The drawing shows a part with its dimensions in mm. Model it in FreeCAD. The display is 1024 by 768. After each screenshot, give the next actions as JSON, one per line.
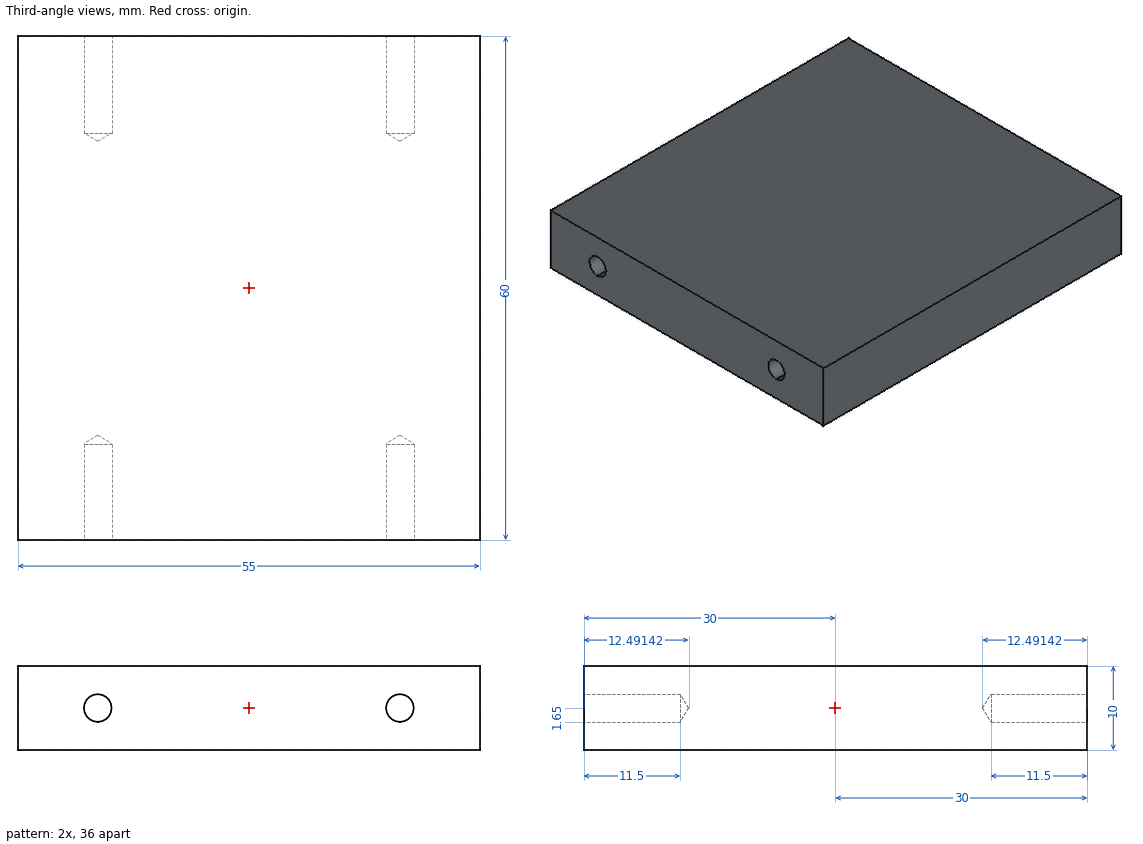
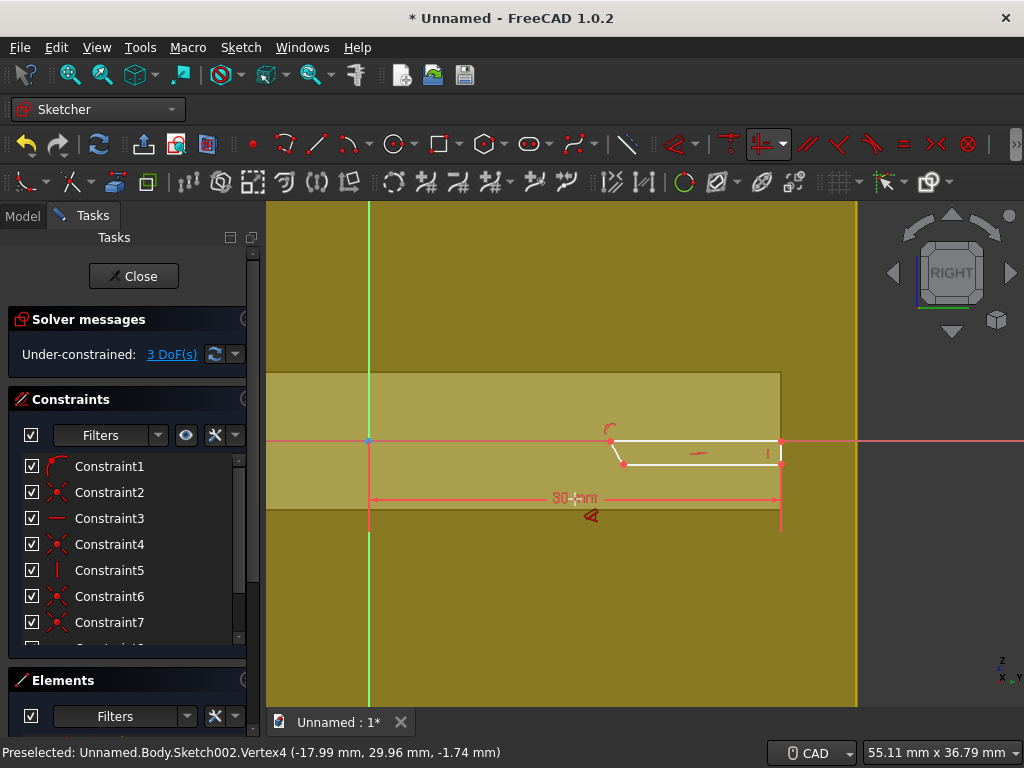
{"action": "left_click", "coordinate": [671, 465]}
{"action": "left_click", "coordinate": [702, 499]}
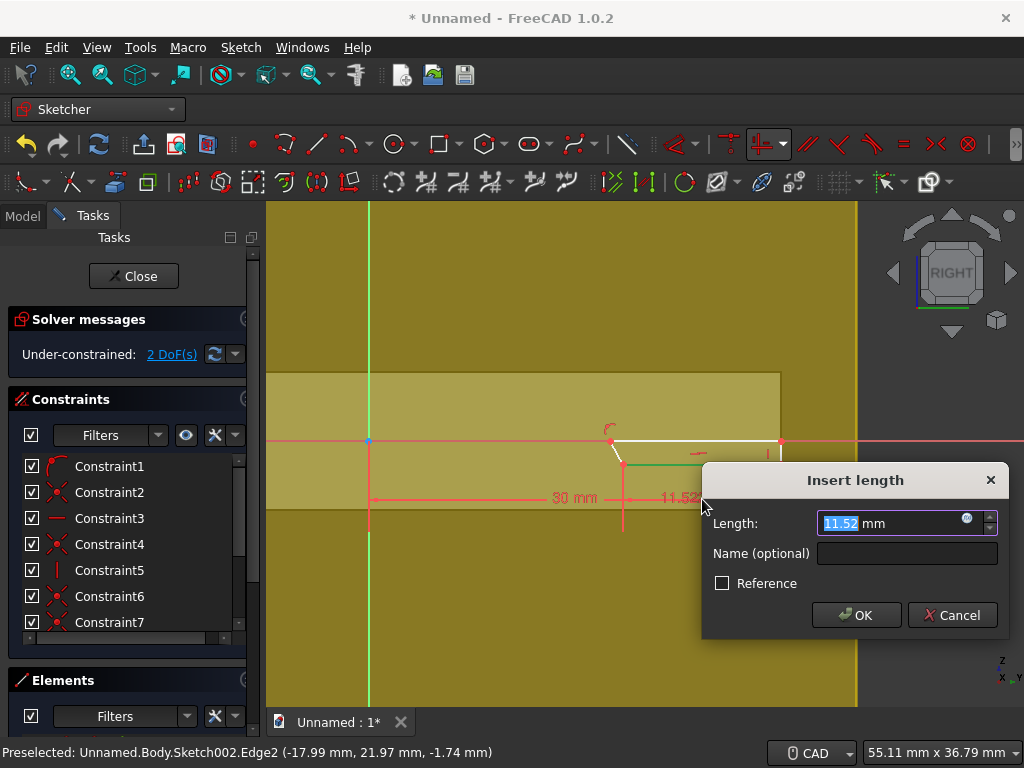
{"action": "type", "text": "11.5"}
{"action": "key", "text": "Return"}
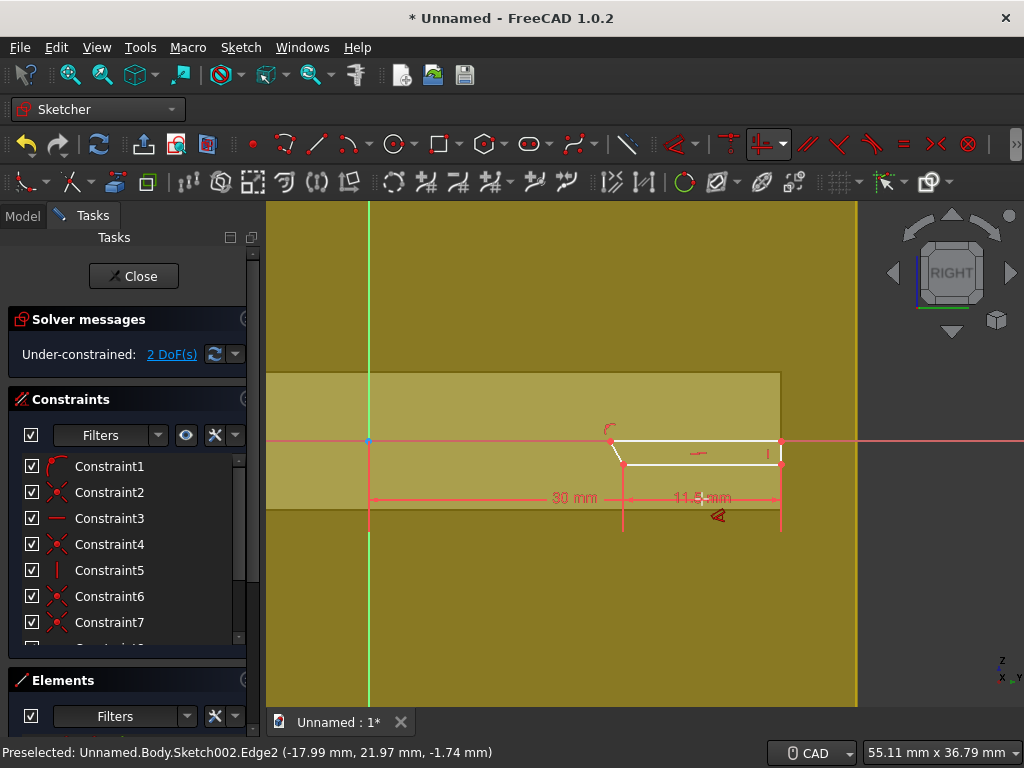
{"action": "scroll", "coordinate": [781, 455], "scroll_direction": "up", "scroll_amount": 3}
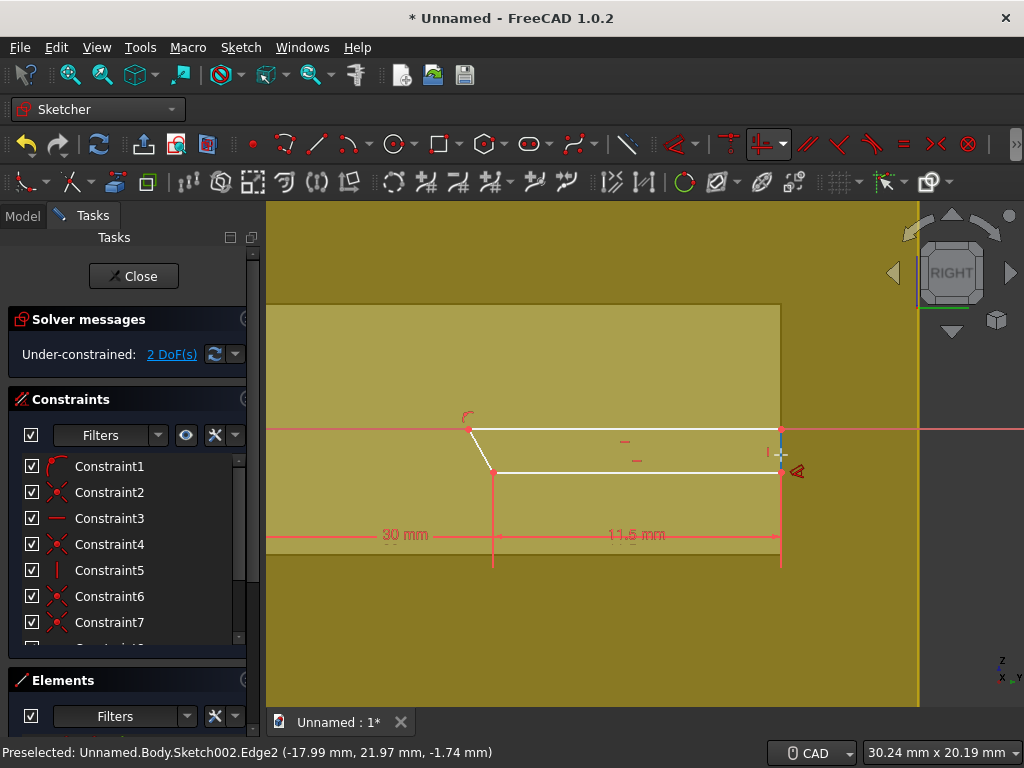
{"action": "left_click", "coordinate": [781, 455]}
{"action": "left_click", "coordinate": [815, 451]}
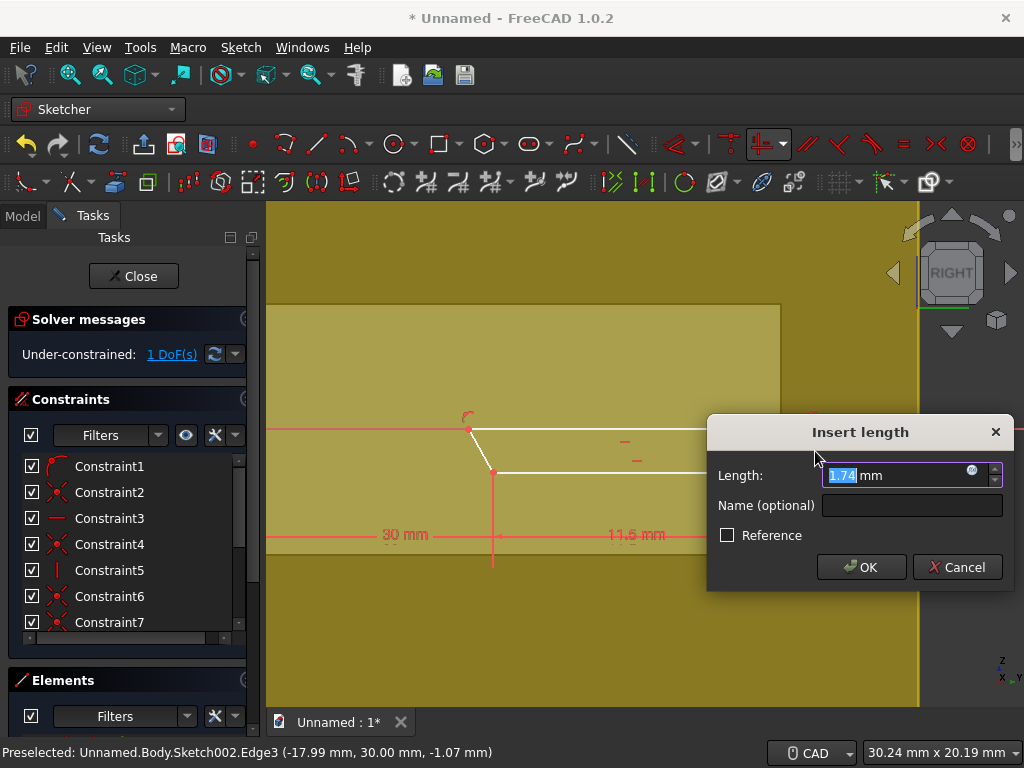
{"action": "type", "text": "1.65"}
{"action": "key", "text": "Return"}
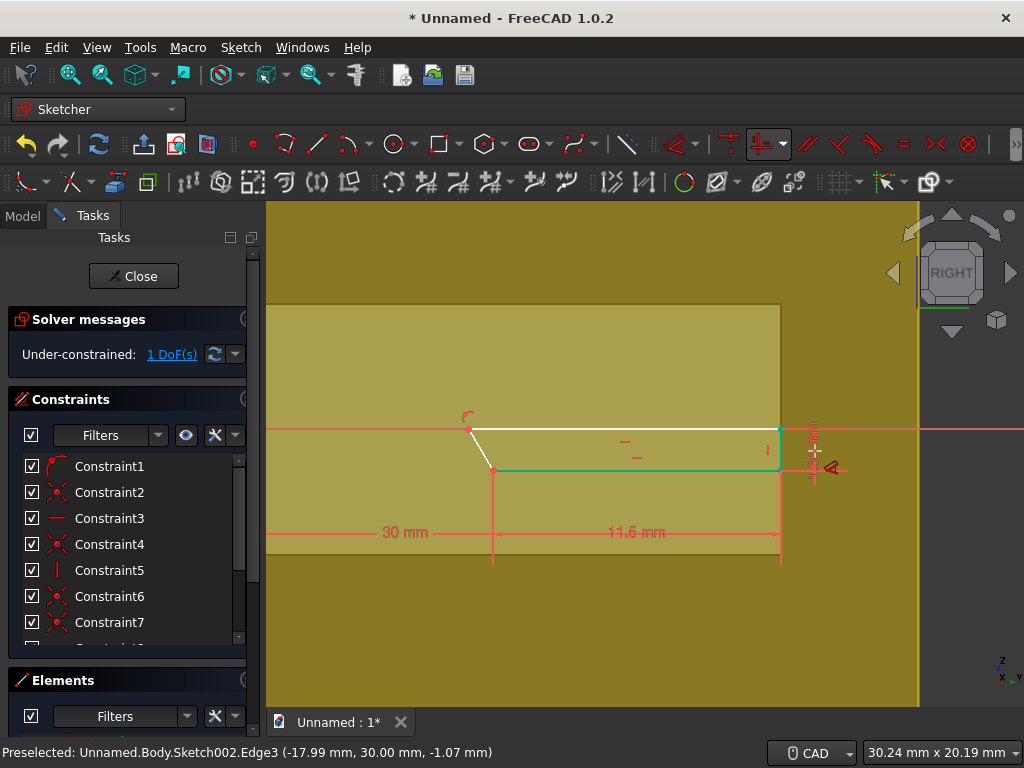
{"action": "left_click", "coordinate": [688, 429]}
{"action": "left_click", "coordinate": [625, 395]}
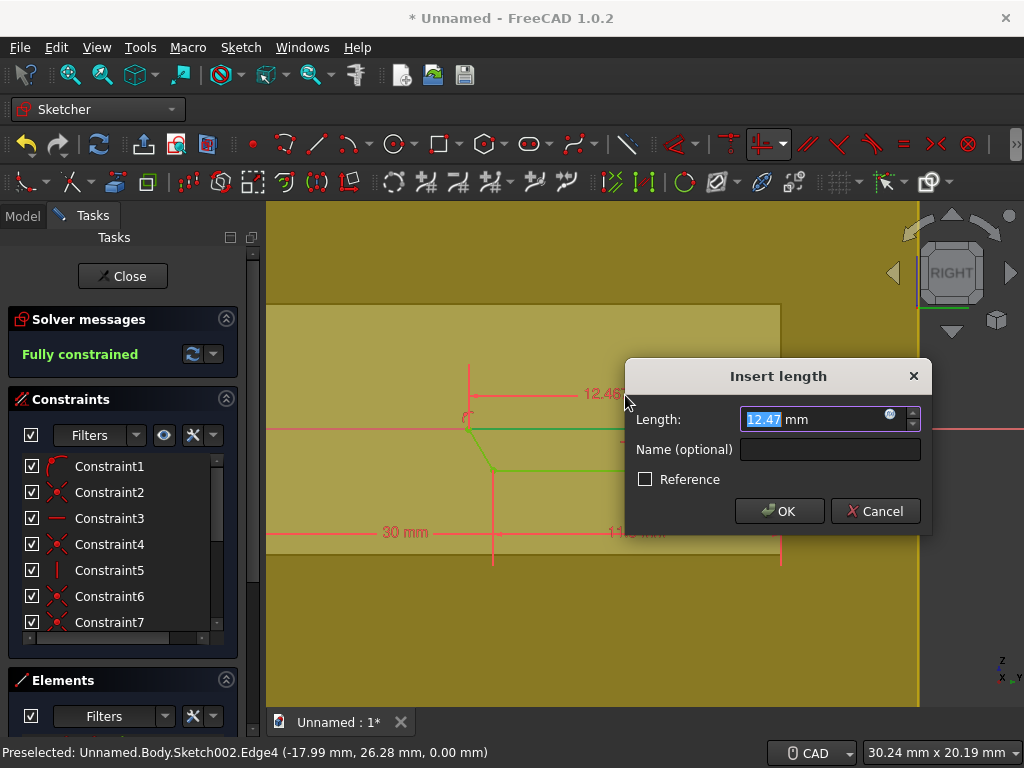
{"action": "type", "text": "12.49142"}
{"action": "key", "text": "Return"}
{"action": "key", "text": "Escape"}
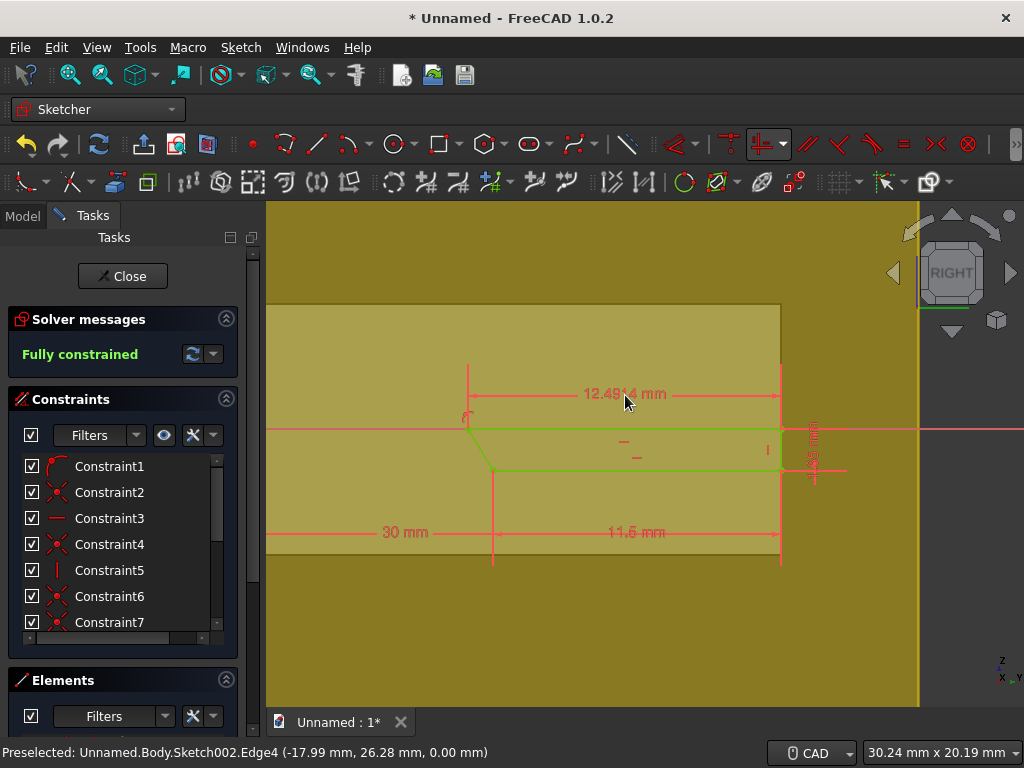
{"action": "left_click", "coordinate": [123, 276]}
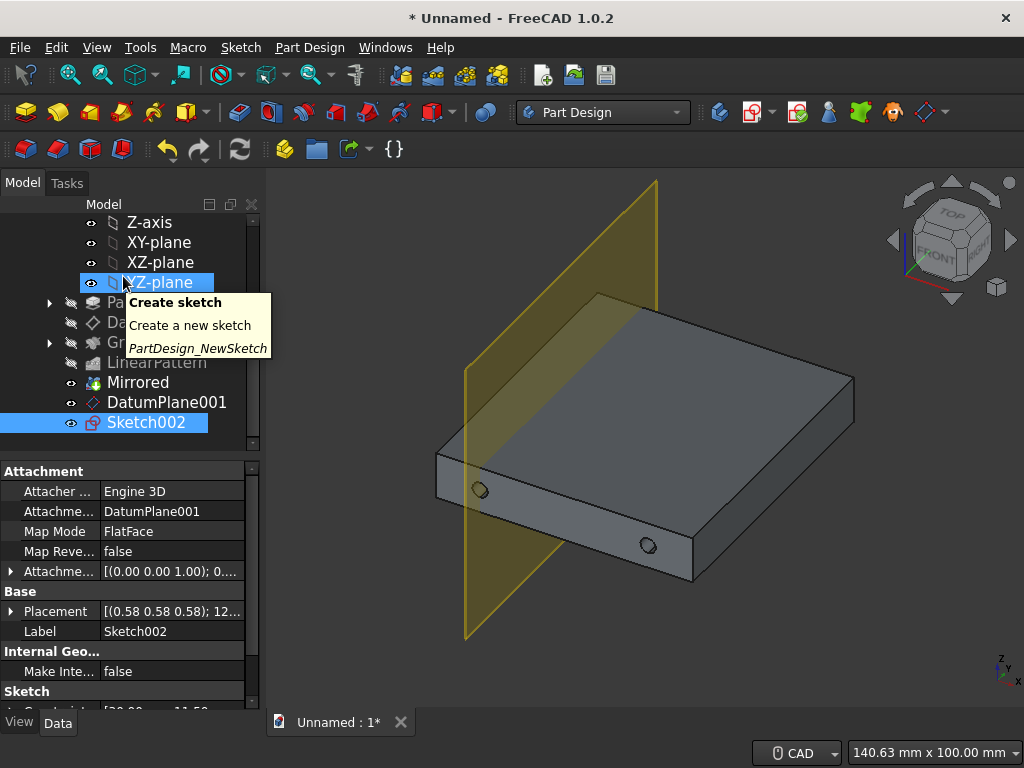
{"action": "left_click", "coordinate": [304, 112]}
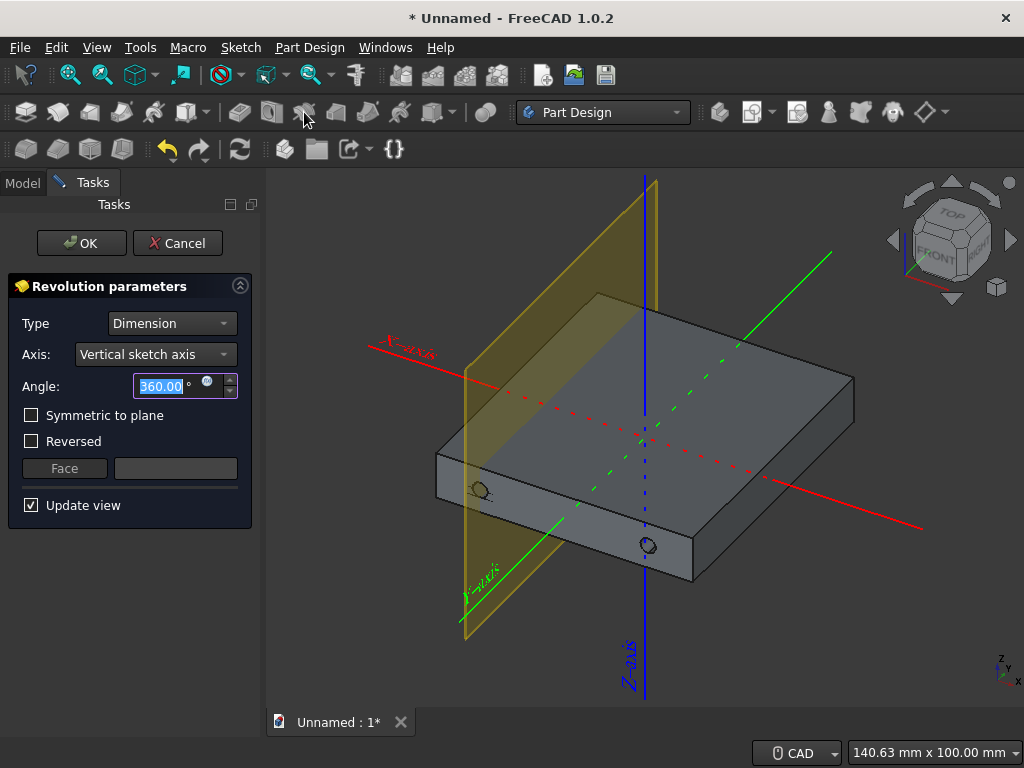
{"action": "left_click", "coordinate": [156, 354]}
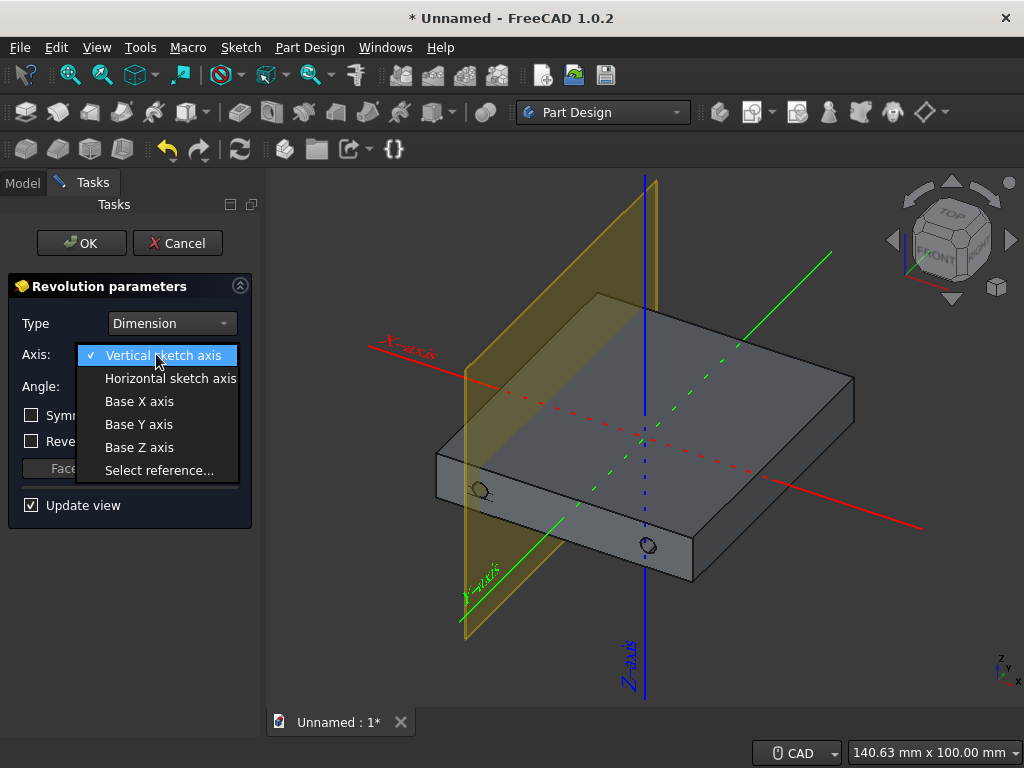
{"action": "left_click", "coordinate": [156, 378]}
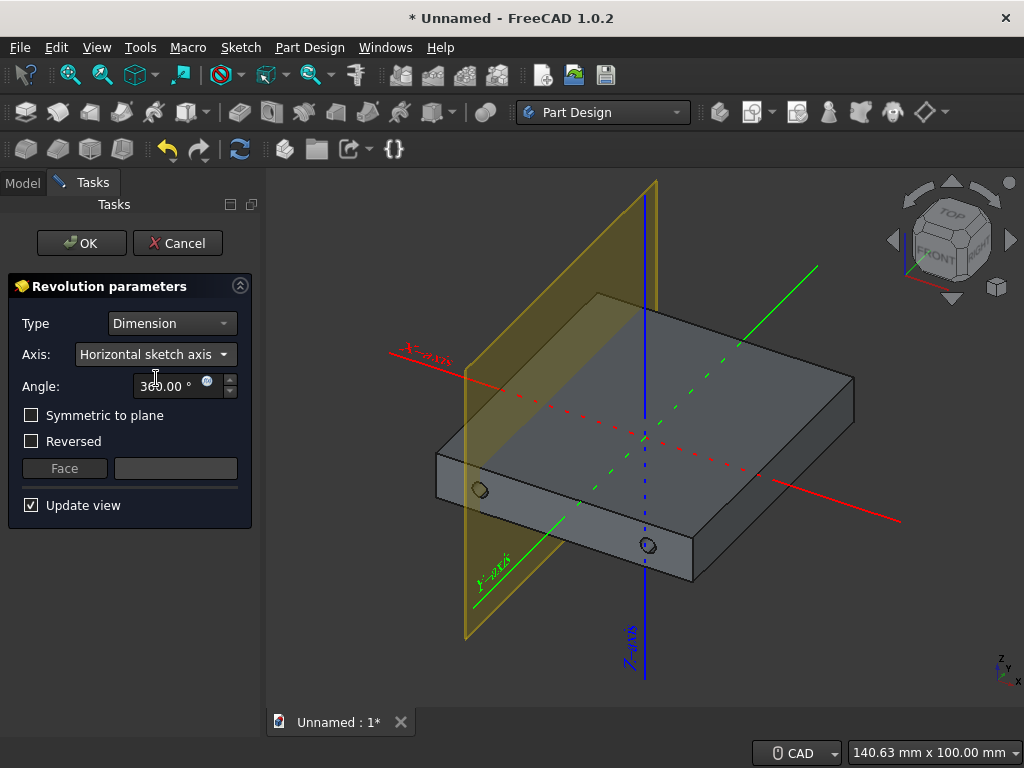
{"action": "left_click", "coordinate": [82, 243]}